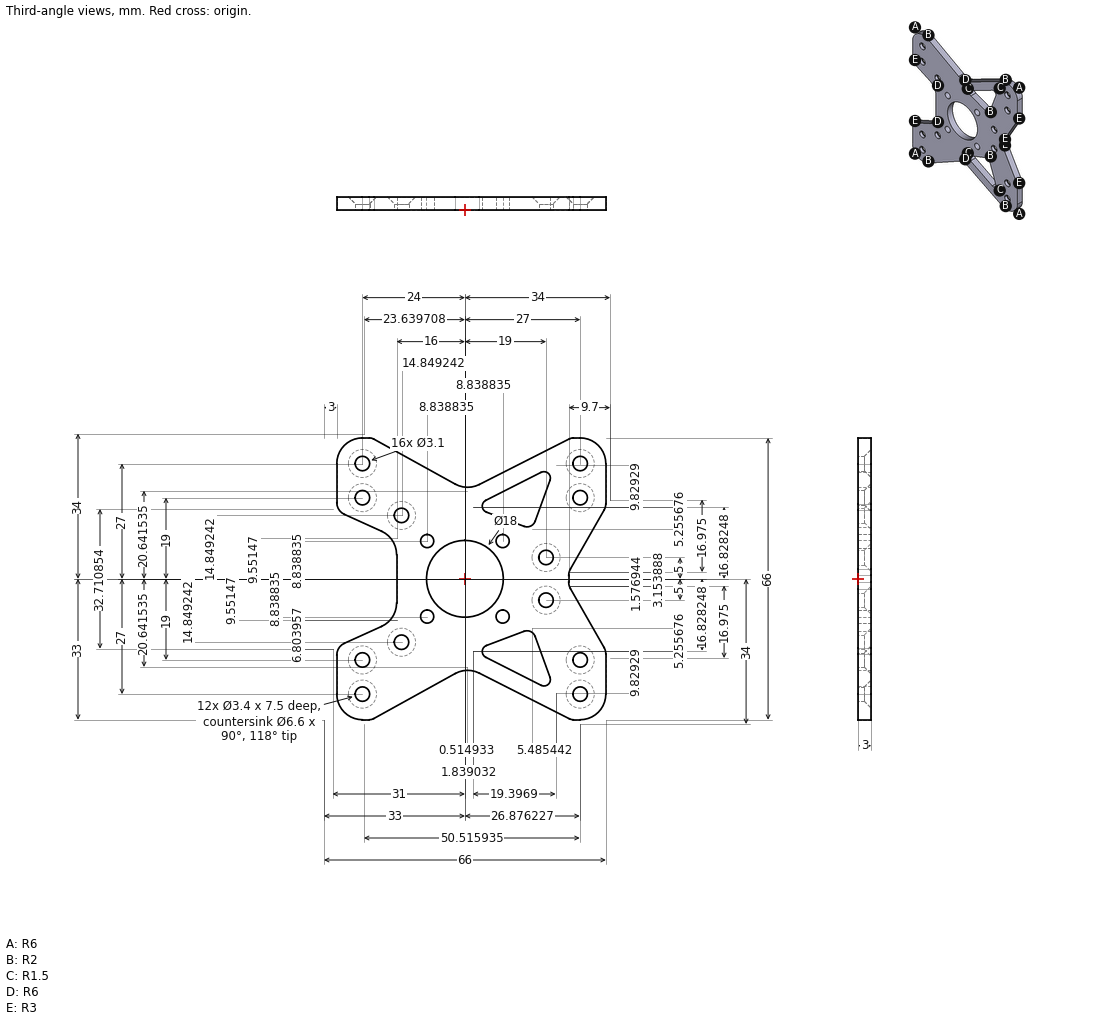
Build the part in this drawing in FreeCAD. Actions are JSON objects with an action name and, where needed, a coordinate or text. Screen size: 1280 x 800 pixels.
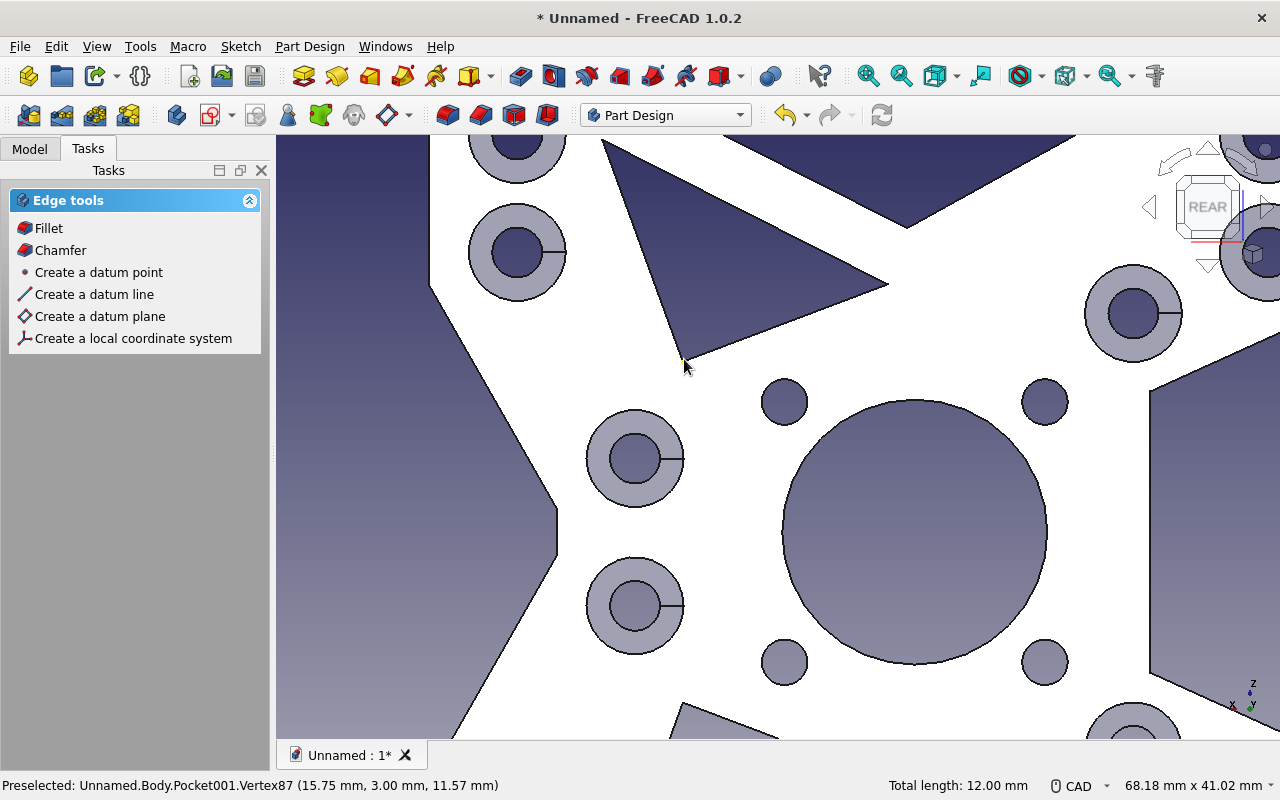
{"action": "key", "text": "v f"}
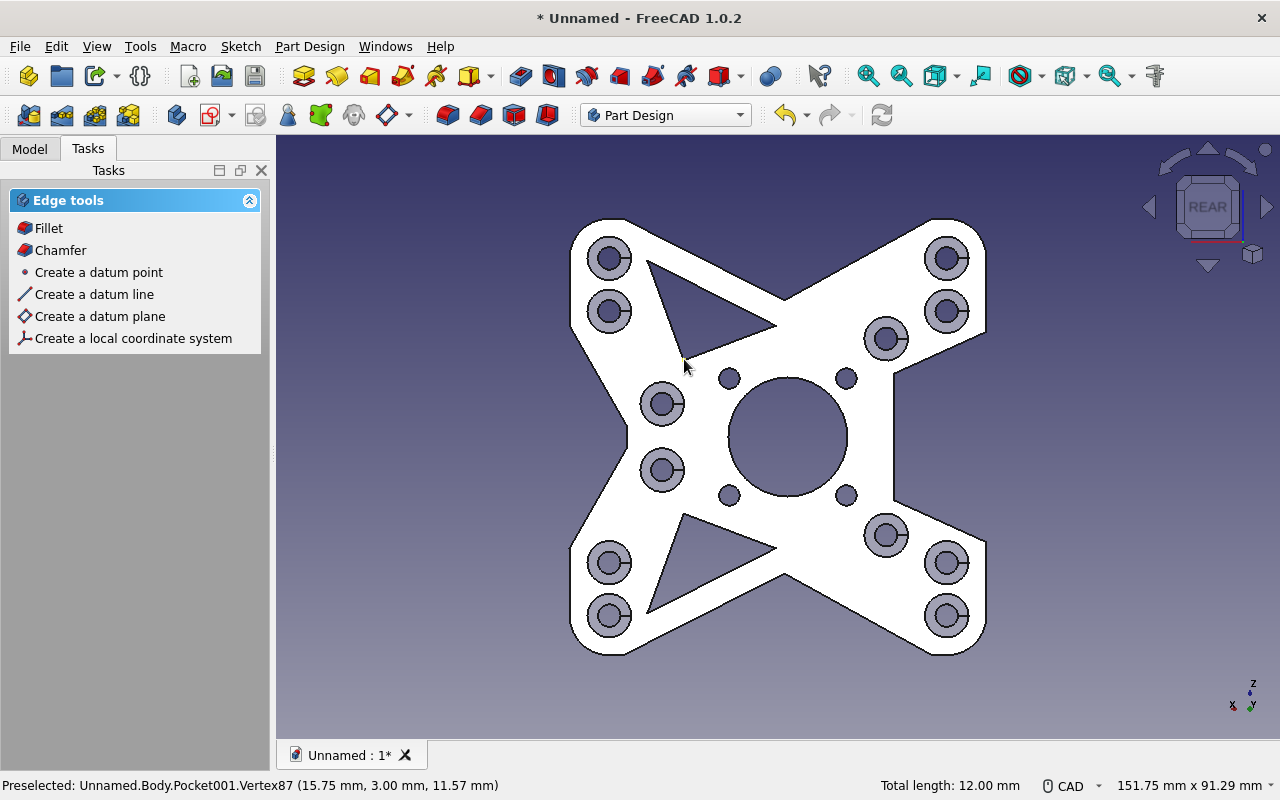
{"action": "key", "text": "6"}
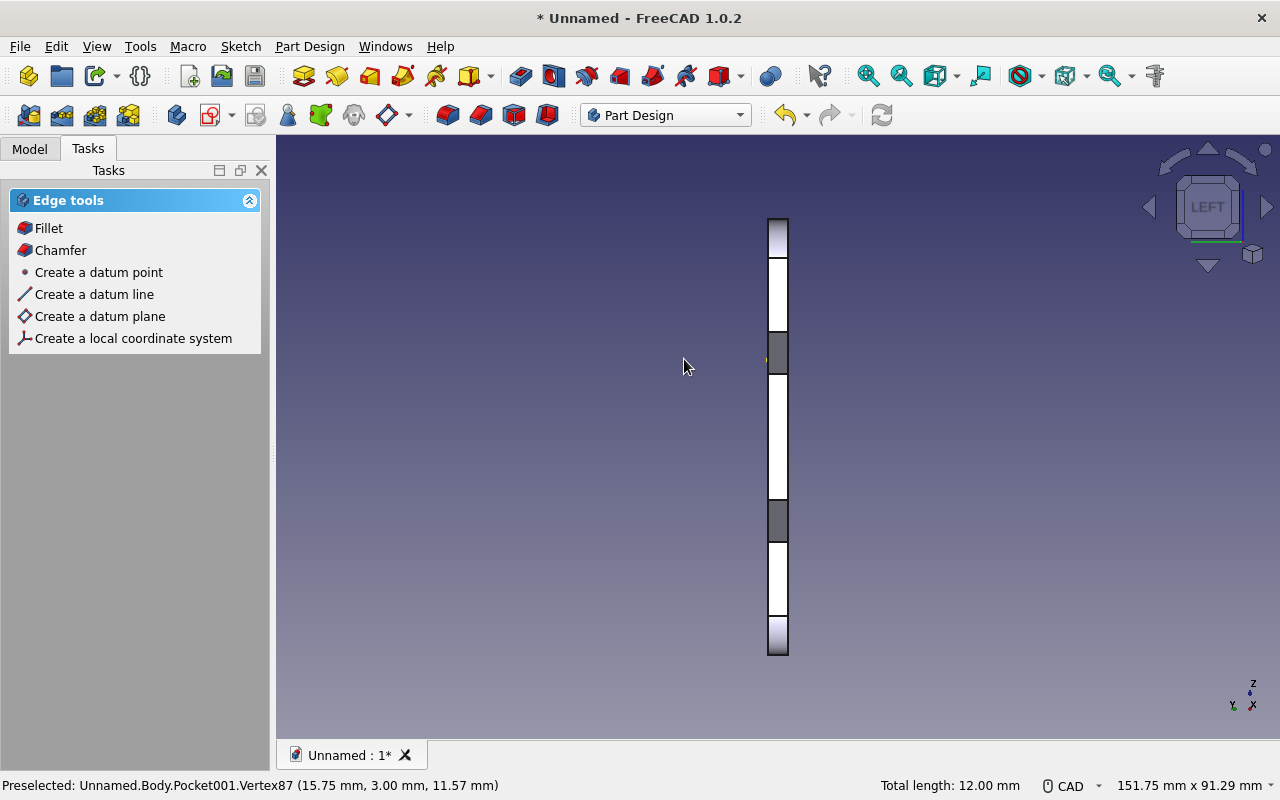
{"action": "scroll", "coordinate": [778, 359], "scroll_direction": "up", "scroll_amount": 4}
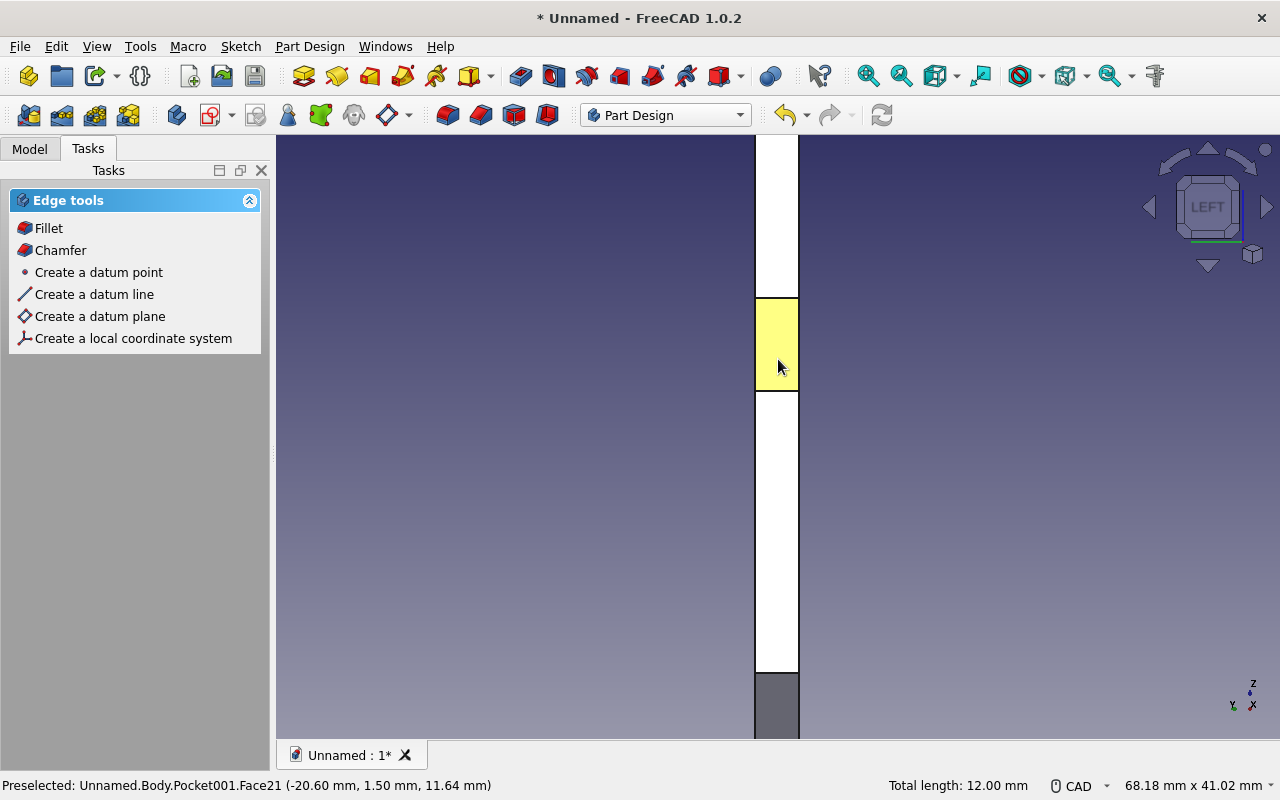
{"action": "key", "text": "v f"}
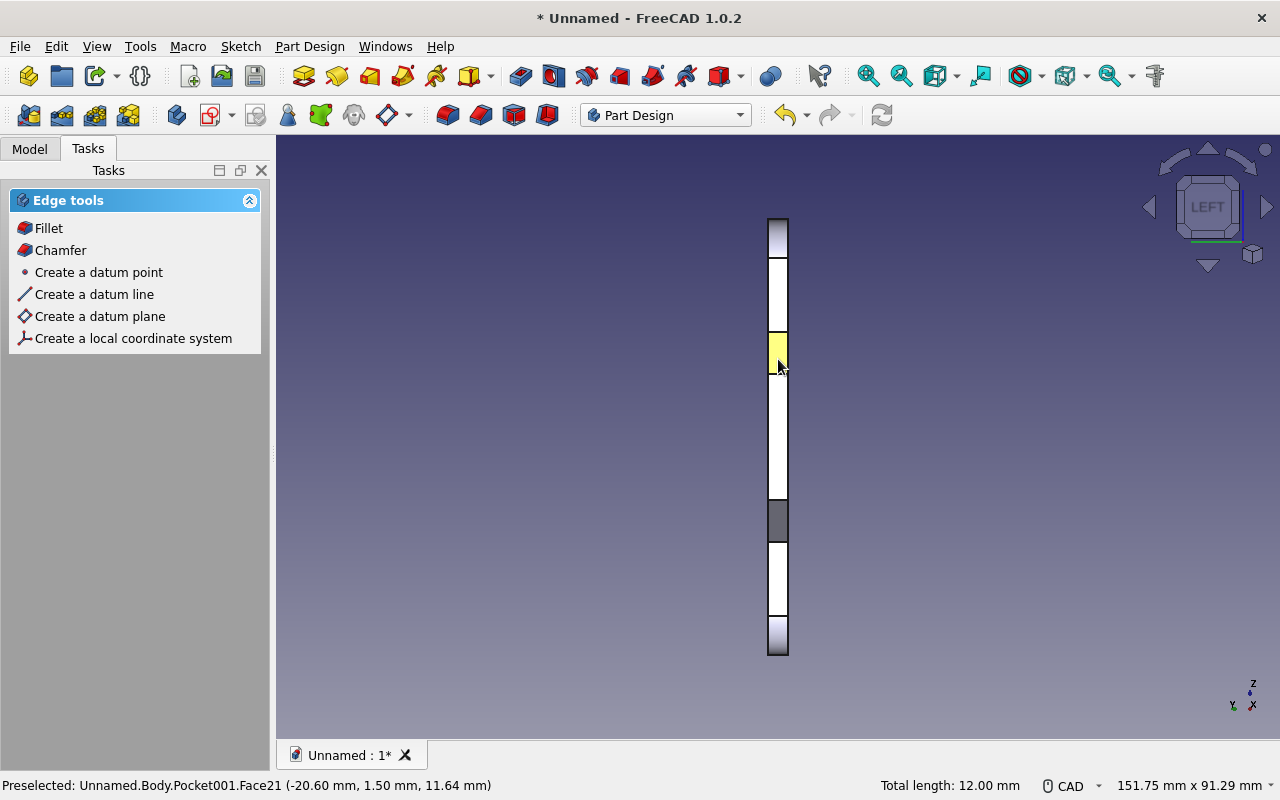
{"action": "key", "text": "v 3"}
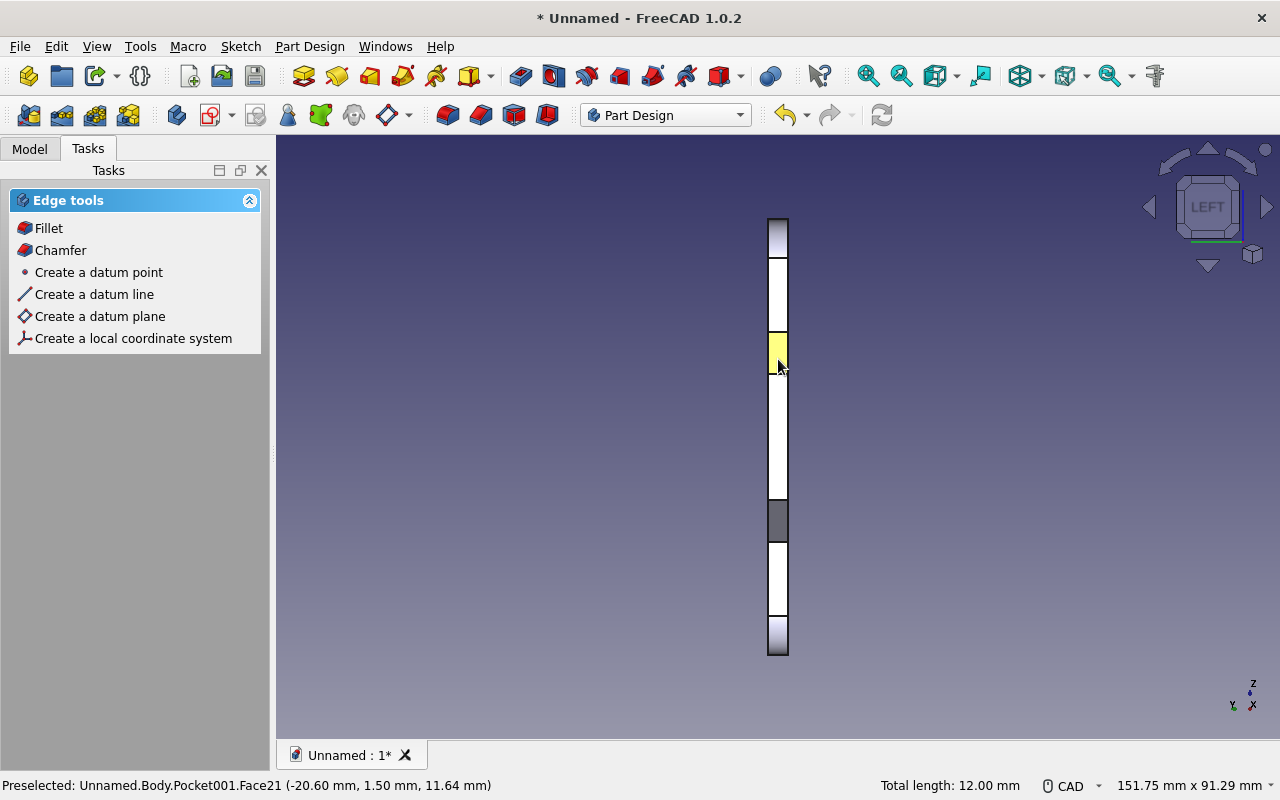
{"action": "key", "text": "0"}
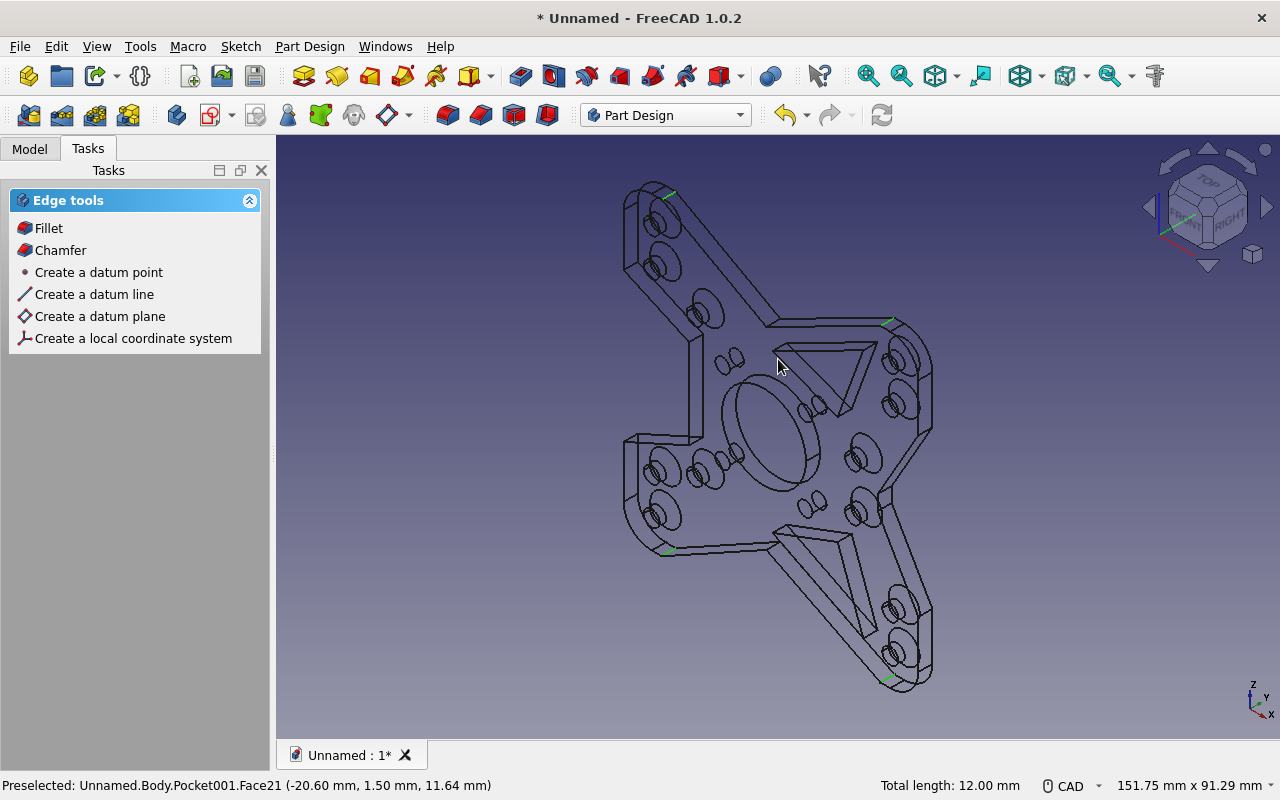
{"action": "left_click", "coordinate": [847, 410], "text": "ctrl"}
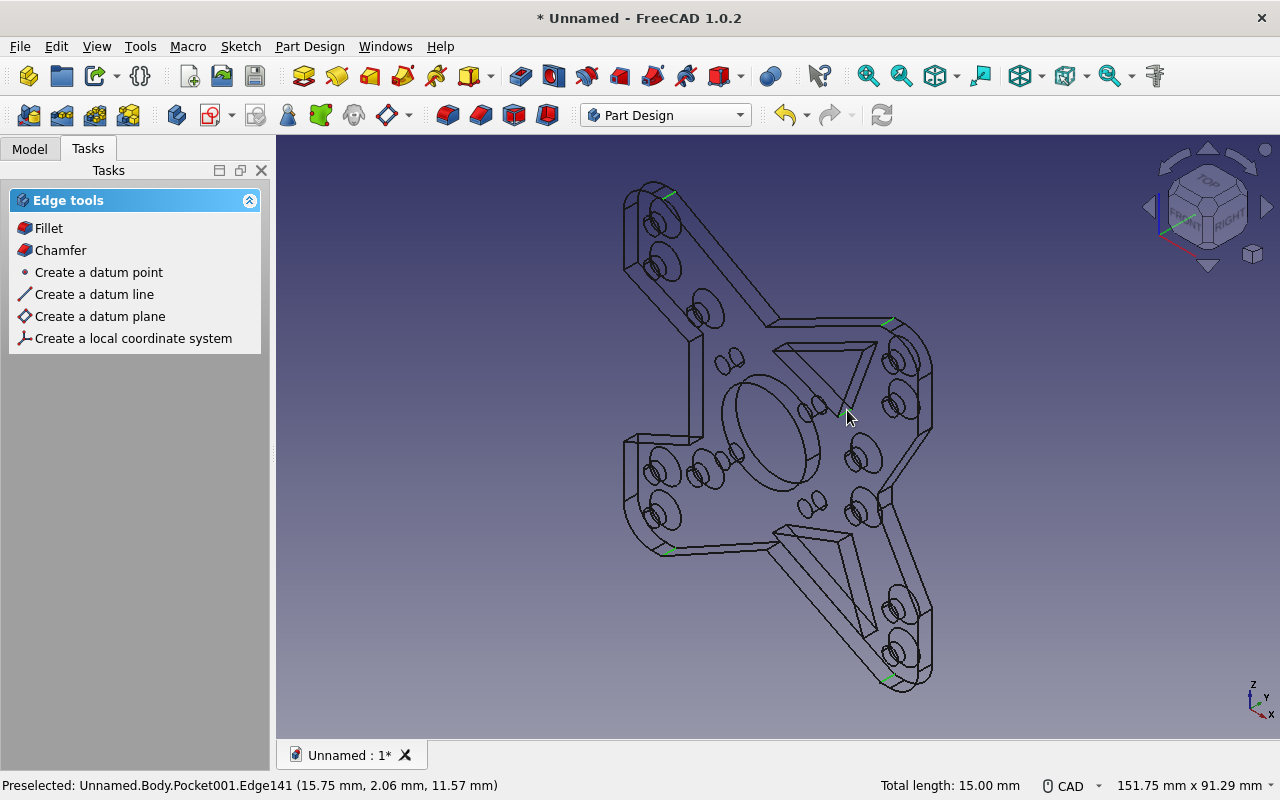
{"action": "left_click", "coordinate": [845, 537], "text": "ctrl"}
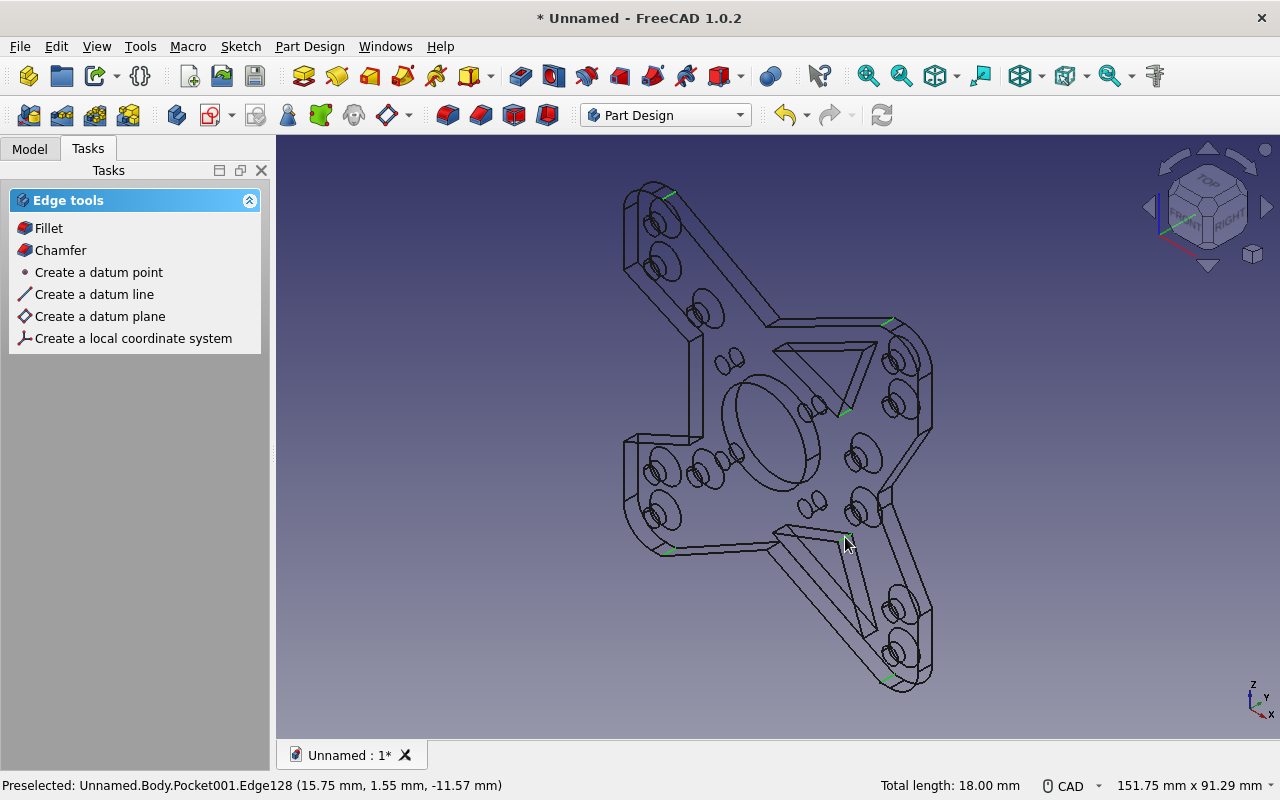
{"action": "key", "text": "v 1"}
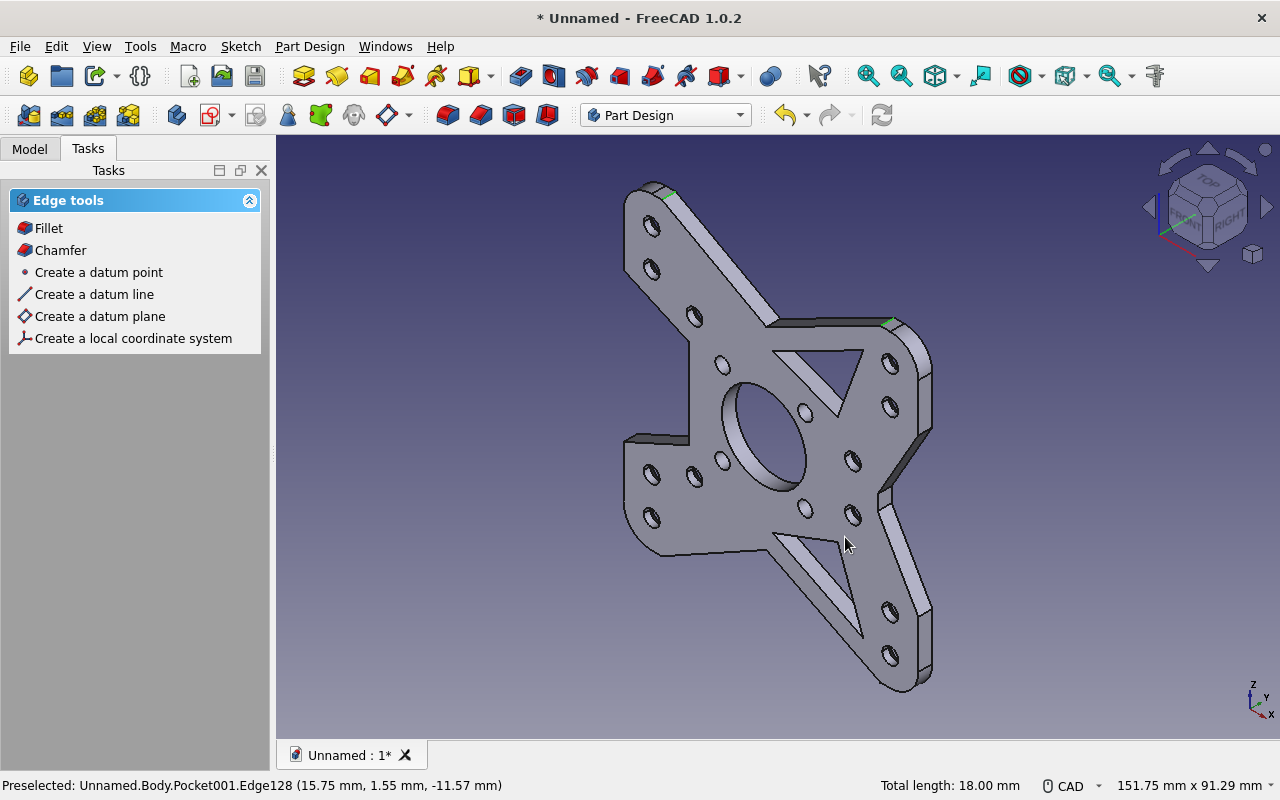
{"action": "left_click", "coordinate": [448, 116]}